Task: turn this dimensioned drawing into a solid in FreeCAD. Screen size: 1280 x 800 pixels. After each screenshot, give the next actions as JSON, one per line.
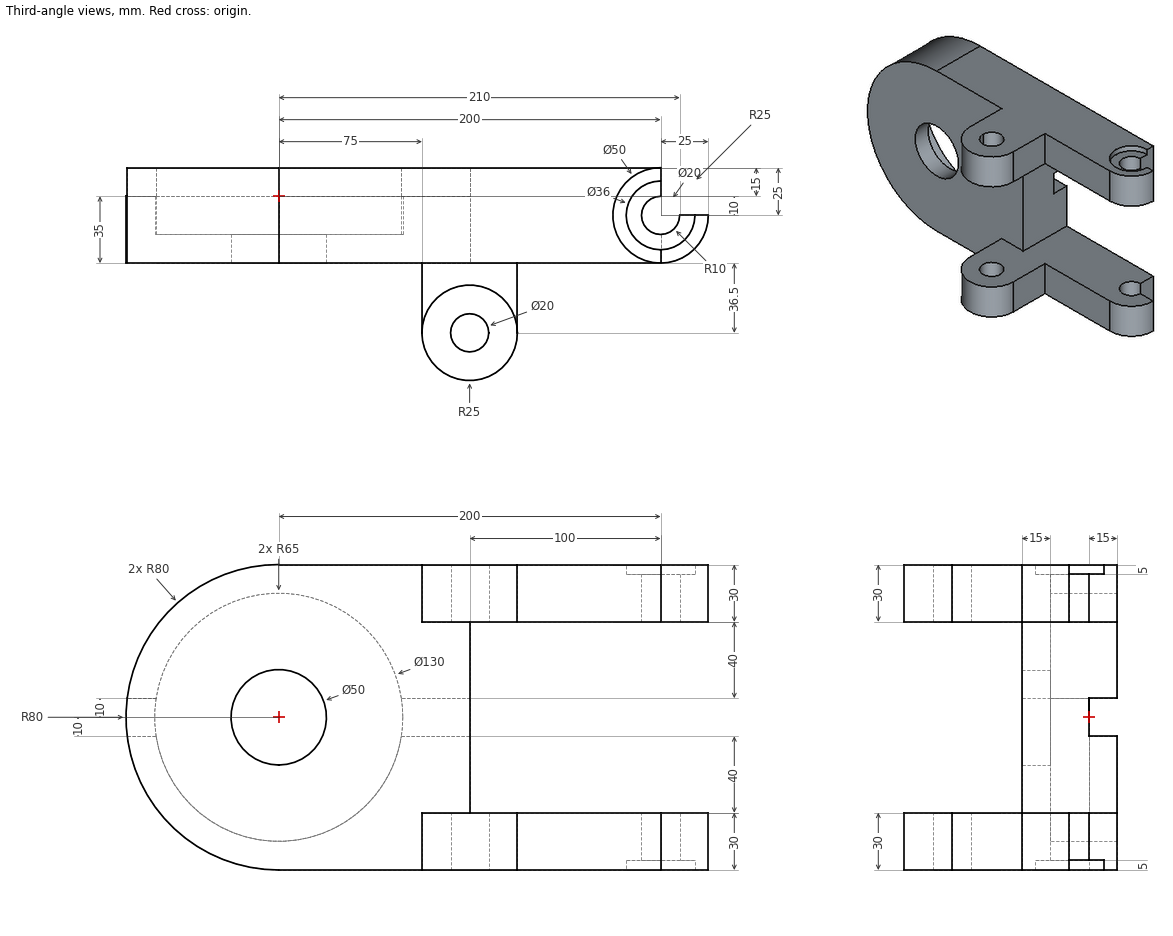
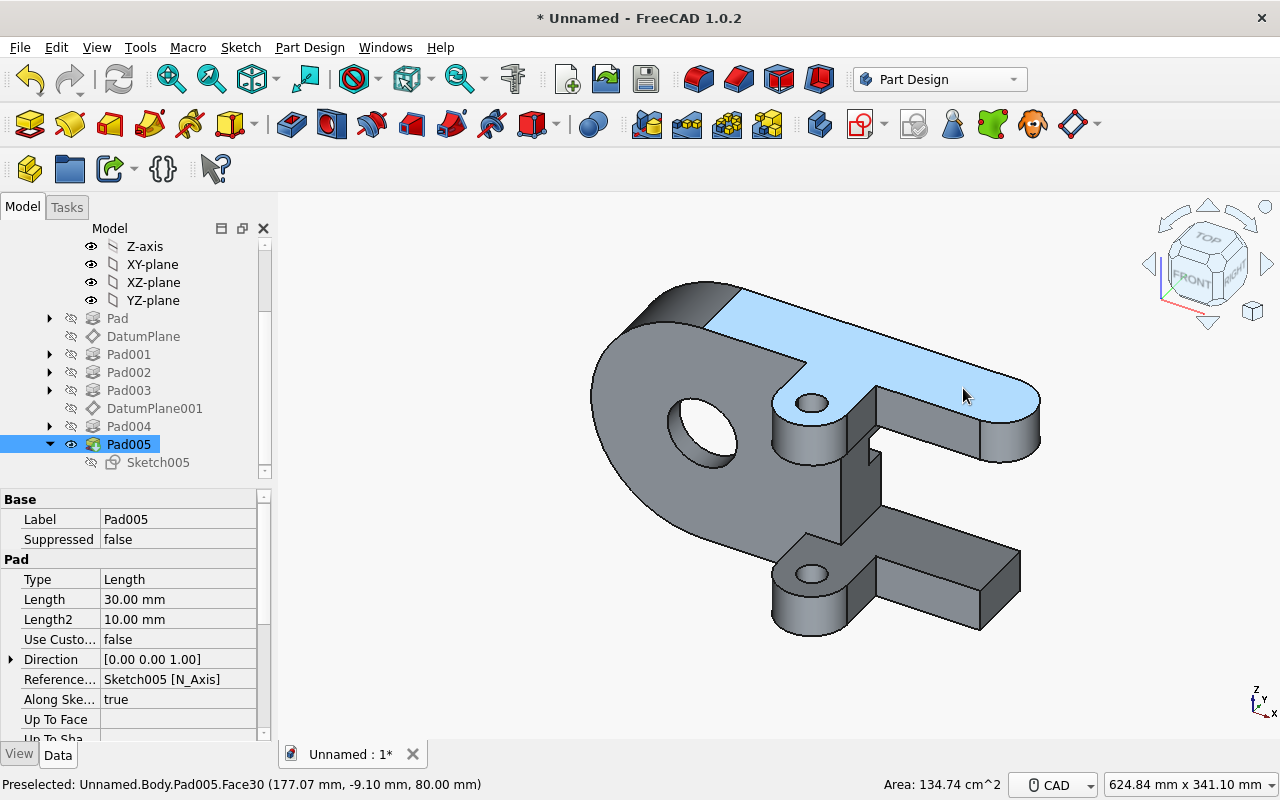
{"action": "left_click", "coordinate": [860, 124]}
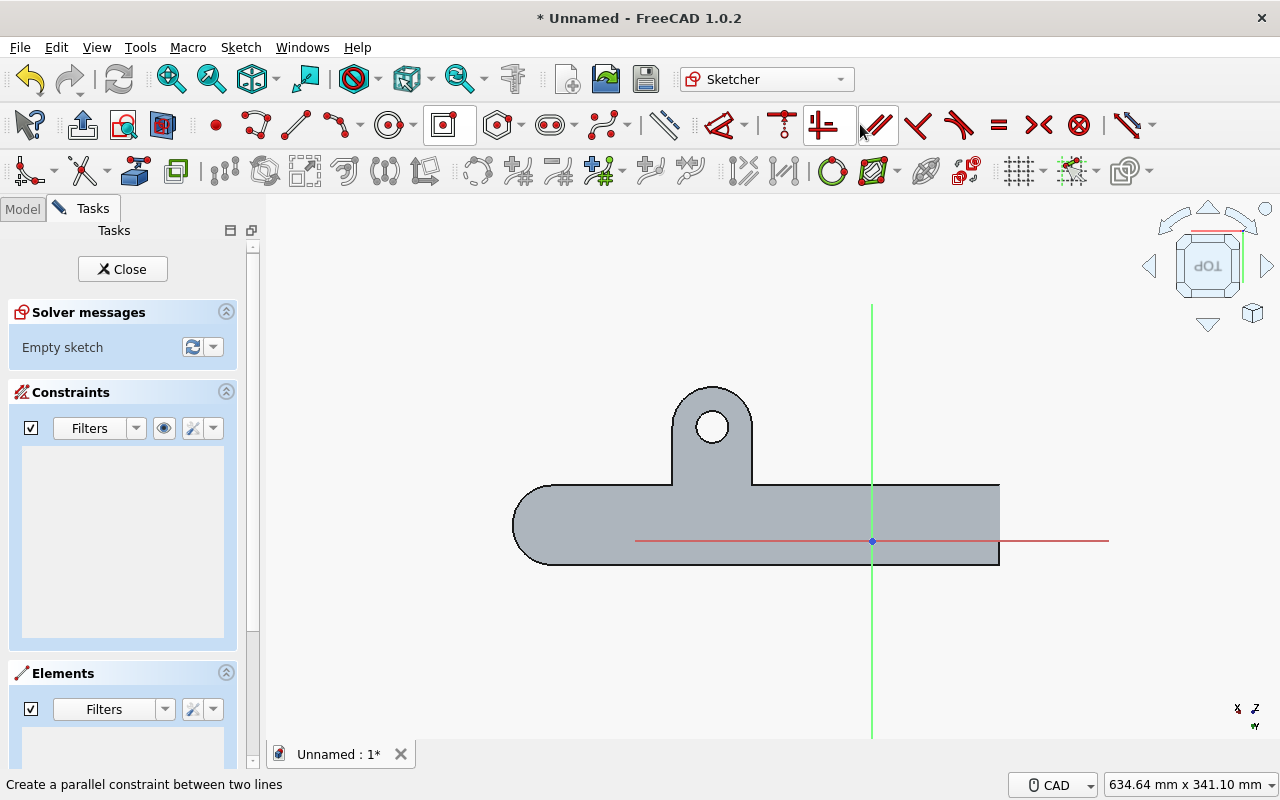
{"action": "scroll", "coordinate": [537, 531], "scroll_direction": "up", "scroll_amount": 12}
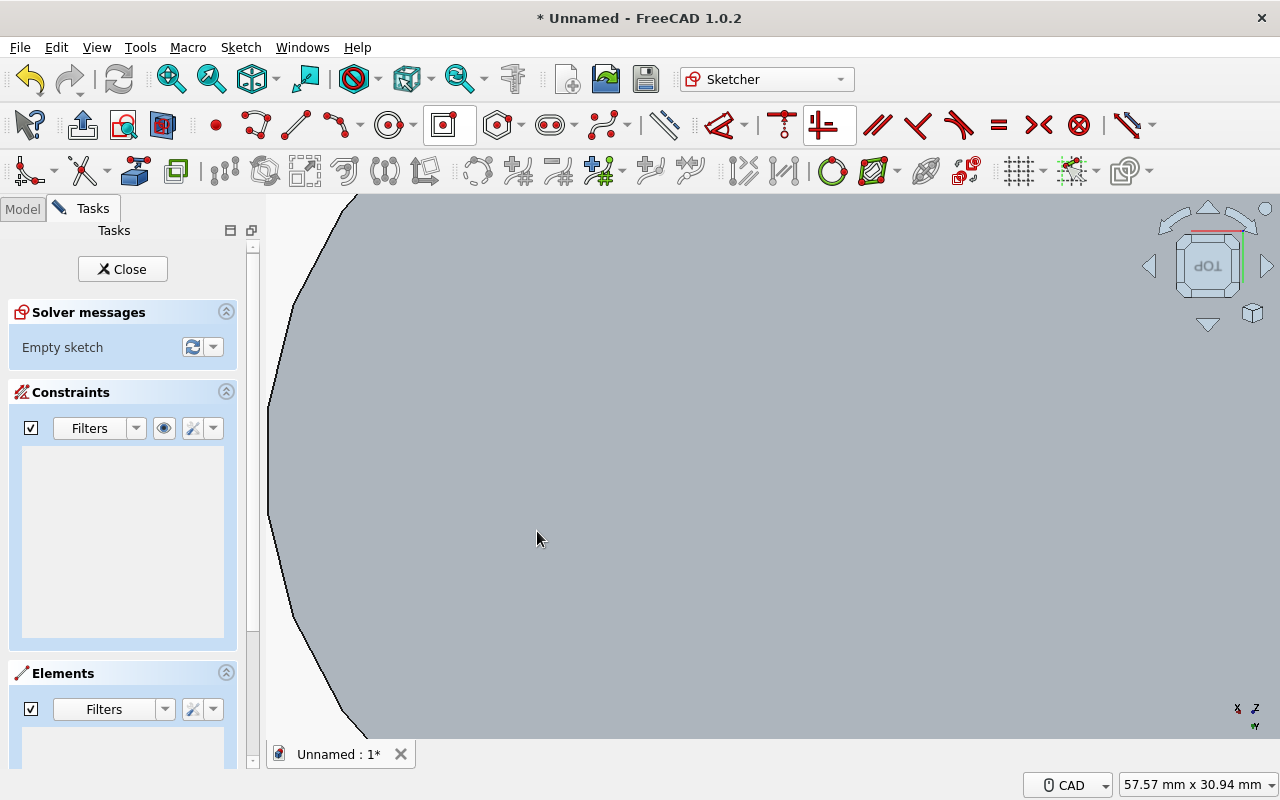
{"action": "left_click", "coordinate": [390, 126]}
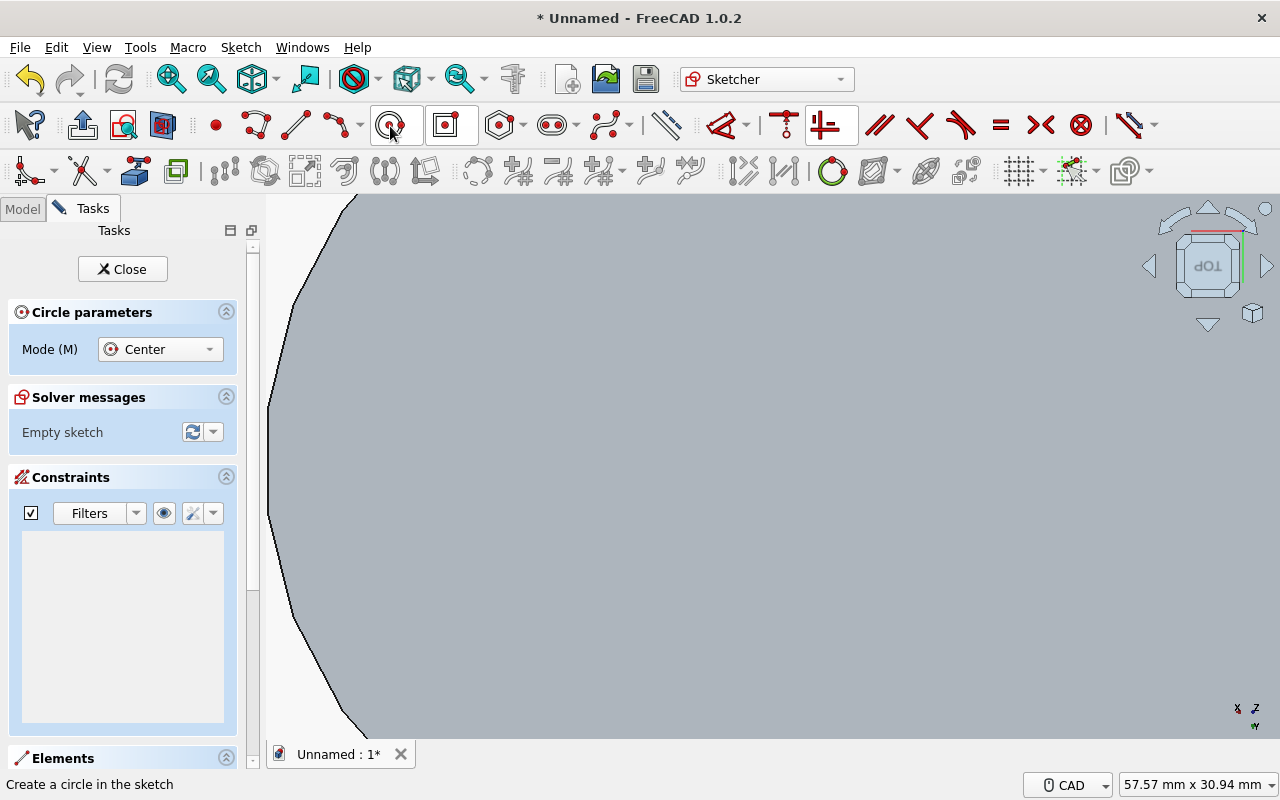
{"action": "left_click", "coordinate": [705, 461]}
{"action": "left_click", "coordinate": [830, 336]}
{"action": "key", "text": "Escape"}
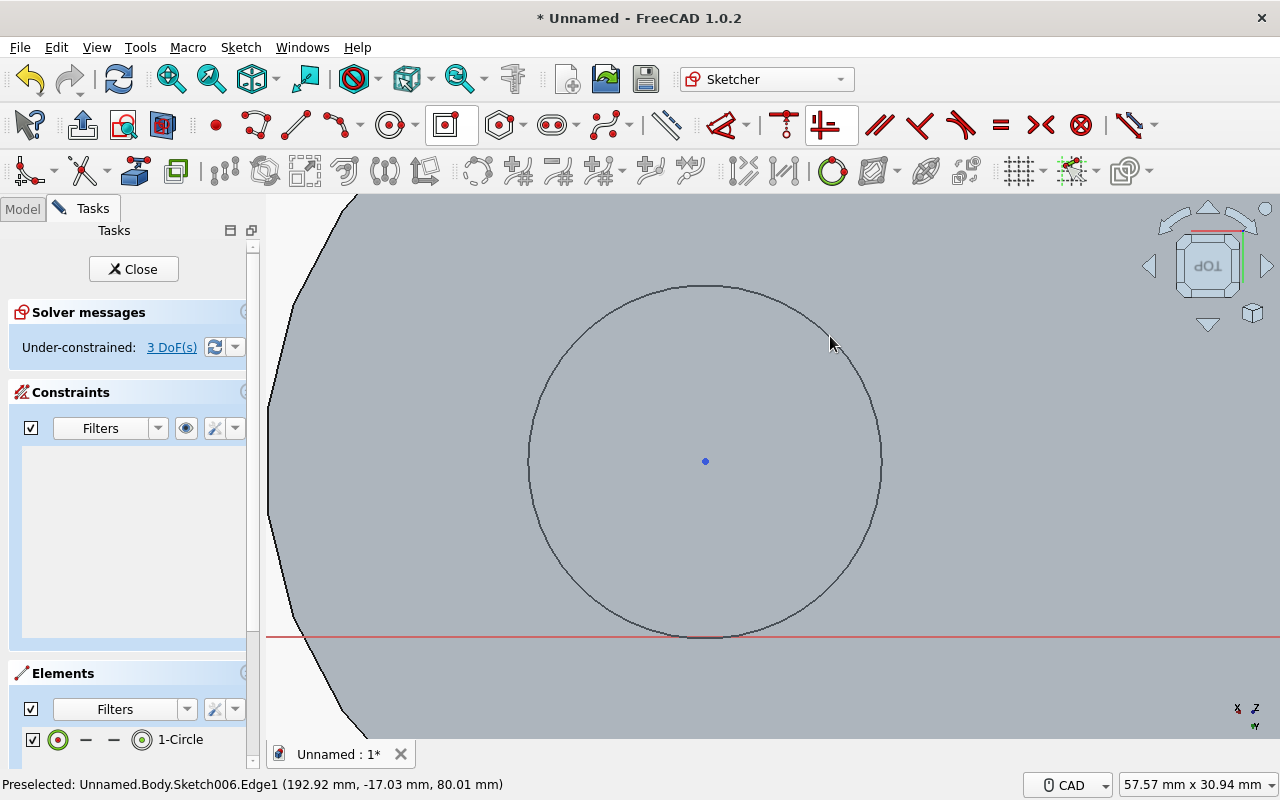
{"action": "left_click", "coordinate": [722, 126]}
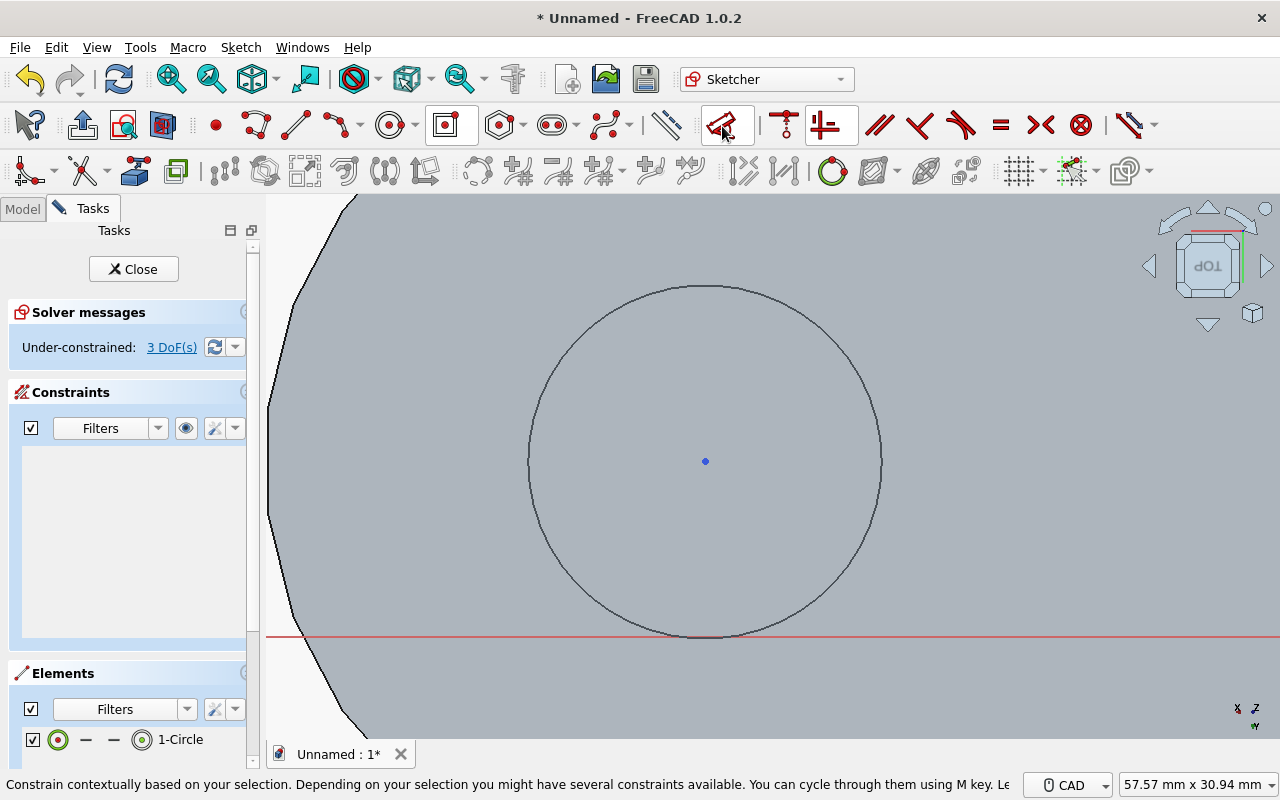
{"action": "left_click", "coordinate": [830, 337]}
{"action": "left_click", "coordinate": [853, 314]}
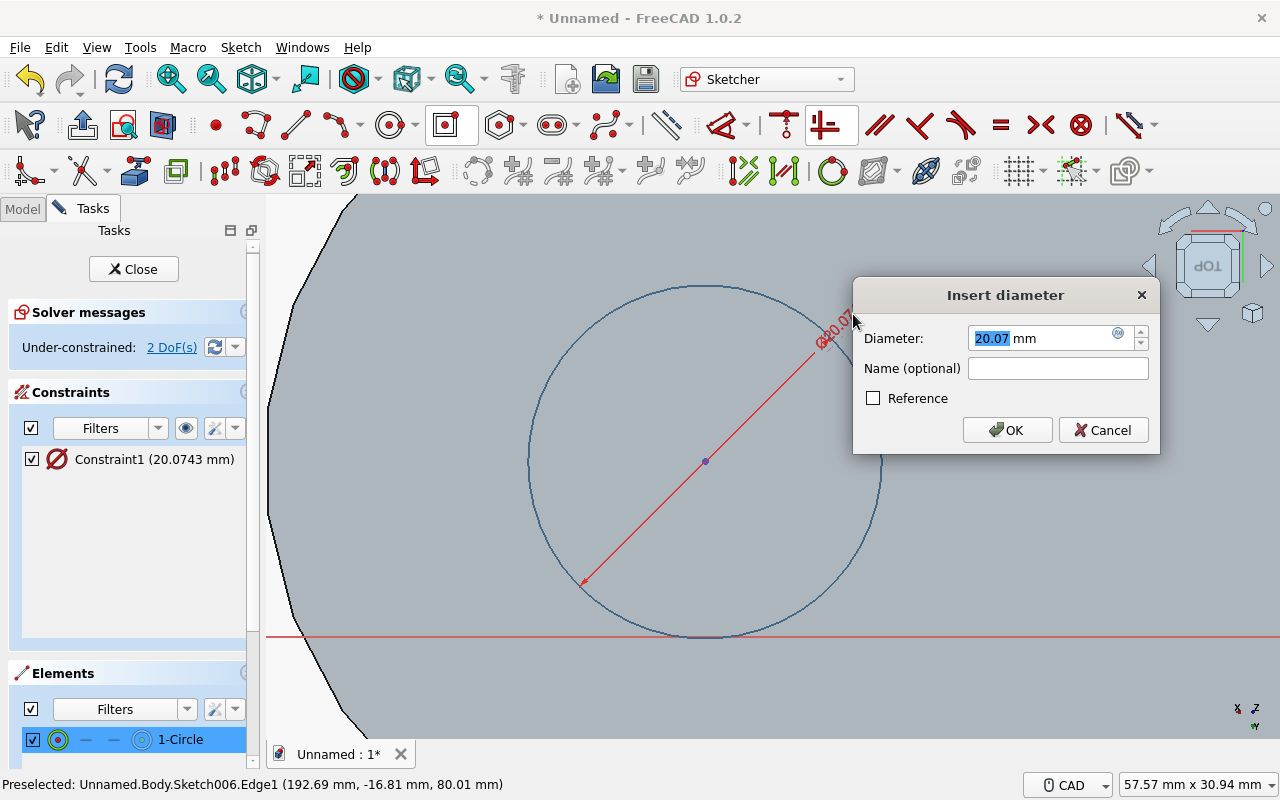
{"action": "type", "text": "20"}
{"action": "key", "text": "Return"}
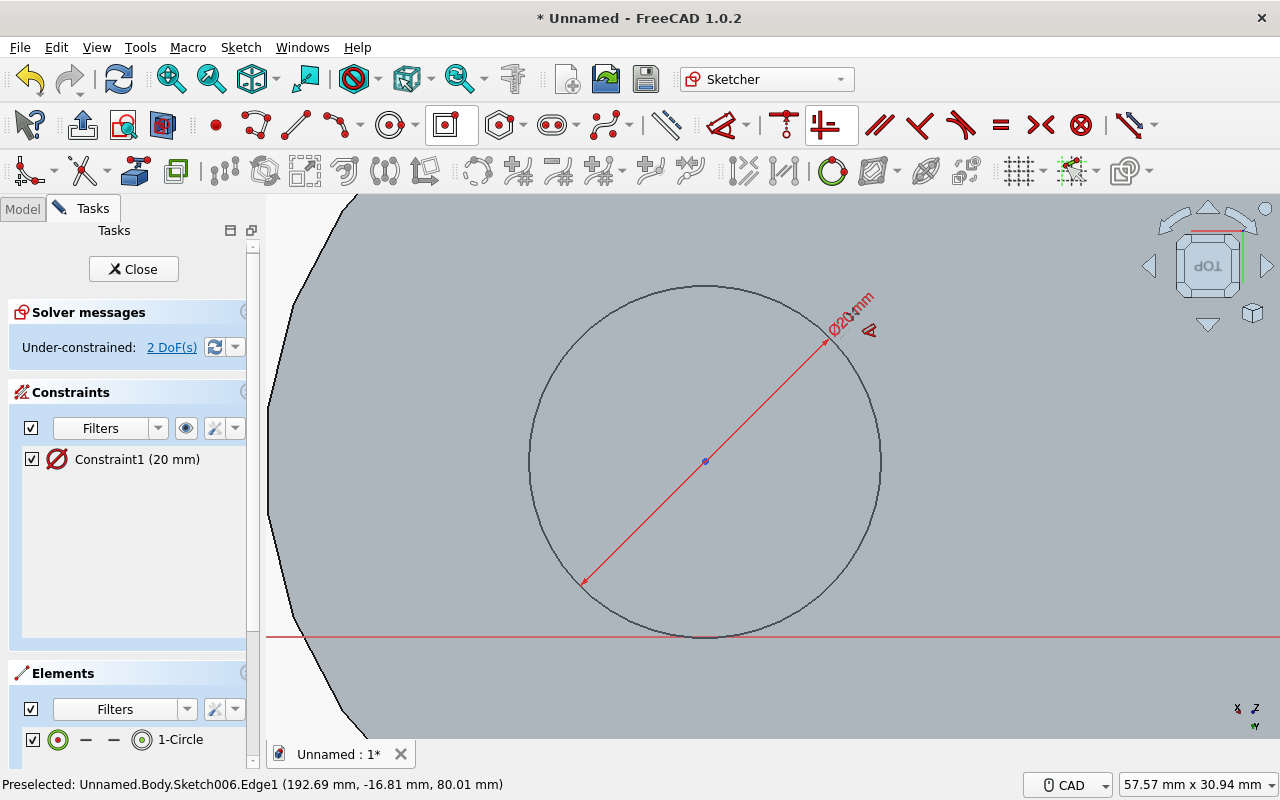
{"action": "left_click", "coordinate": [705, 462]}
{"action": "left_click", "coordinate": [671, 550]}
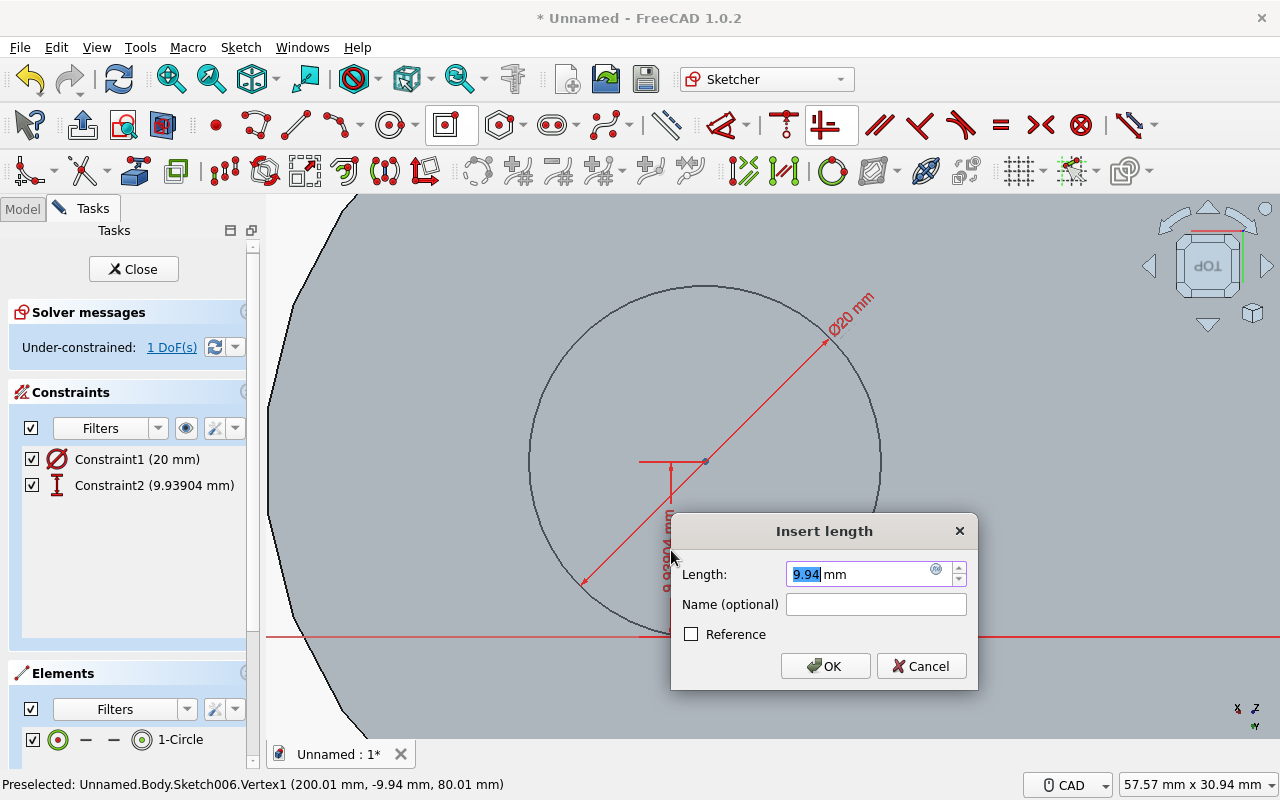
{"action": "type", "text": "10"}
{"action": "key", "text": "Return"}